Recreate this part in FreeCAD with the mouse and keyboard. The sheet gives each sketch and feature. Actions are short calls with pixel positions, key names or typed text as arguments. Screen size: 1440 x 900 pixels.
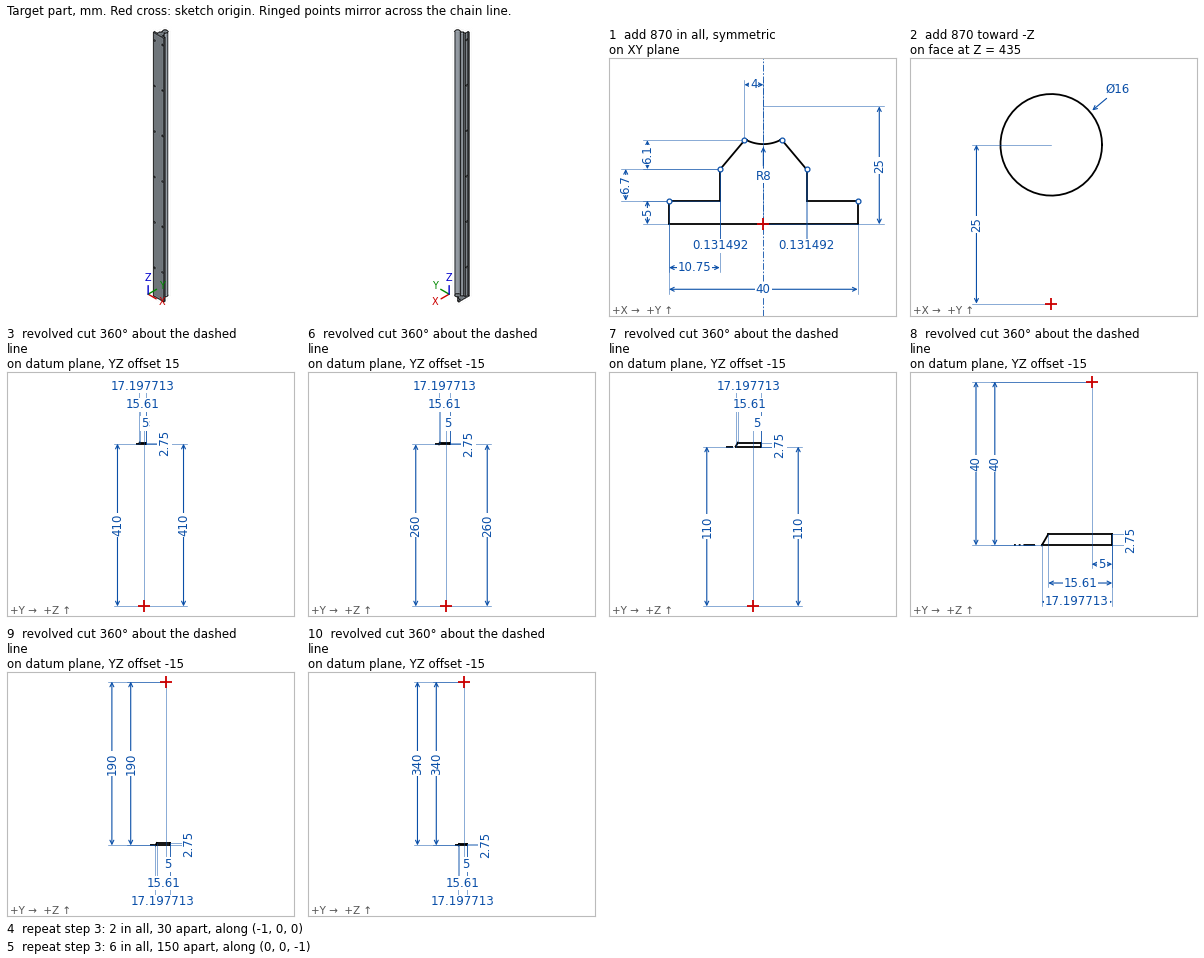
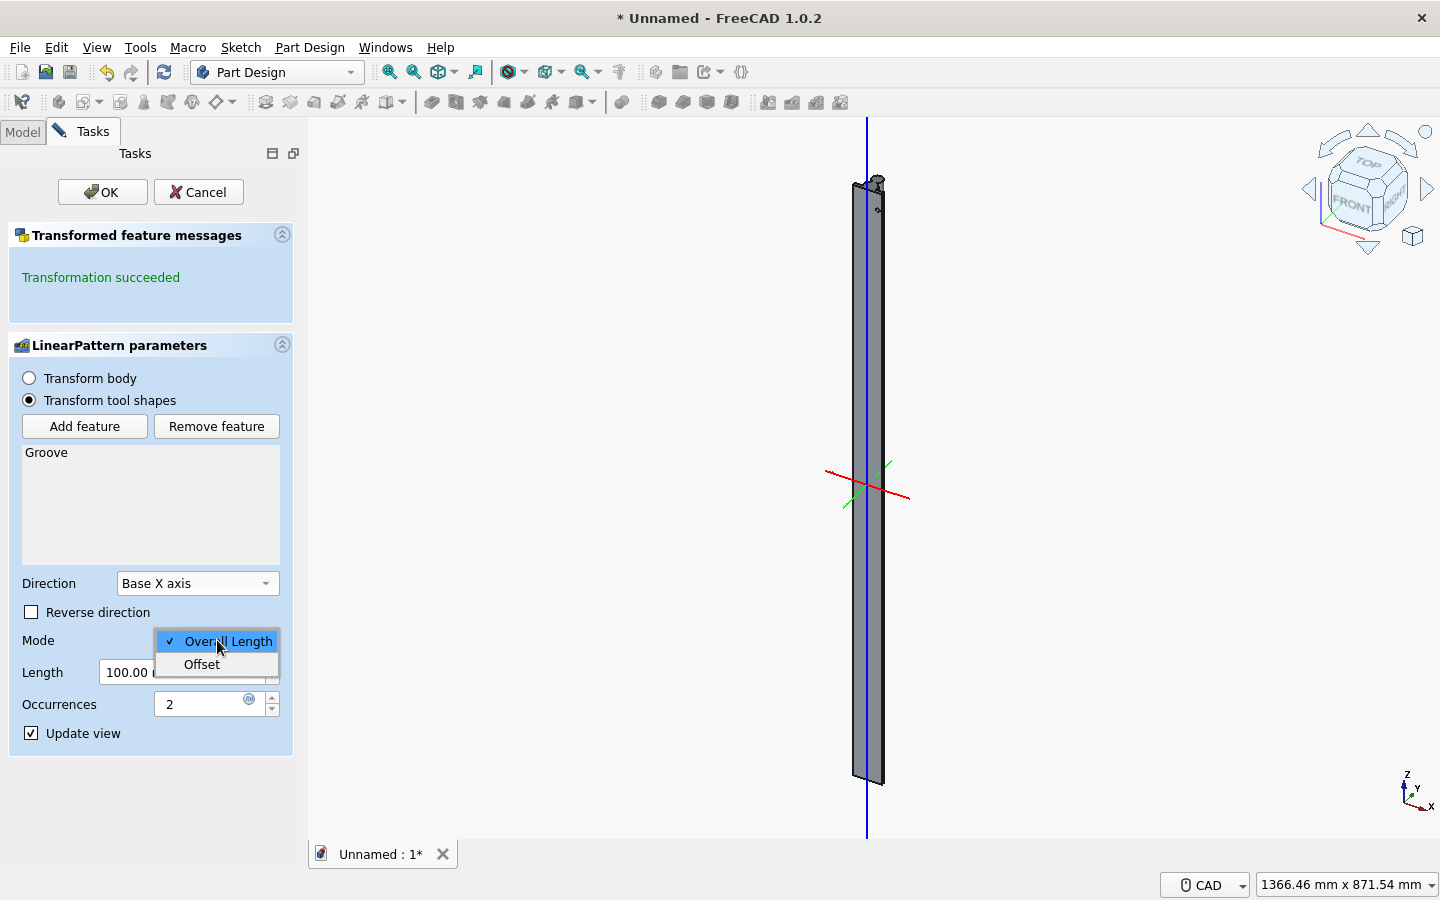
click(216, 664)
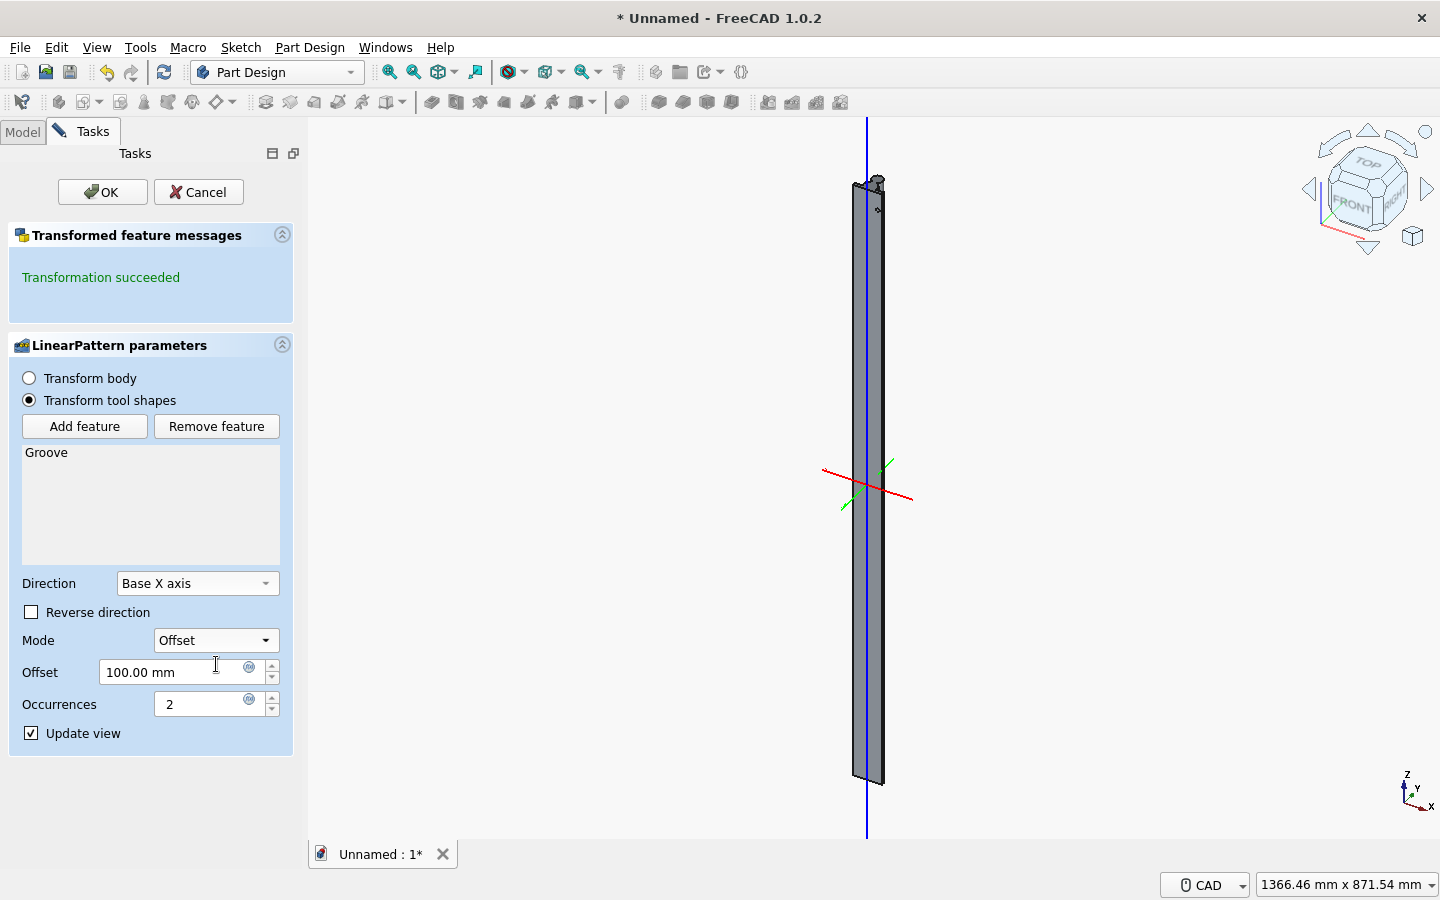
triple_click(182, 672)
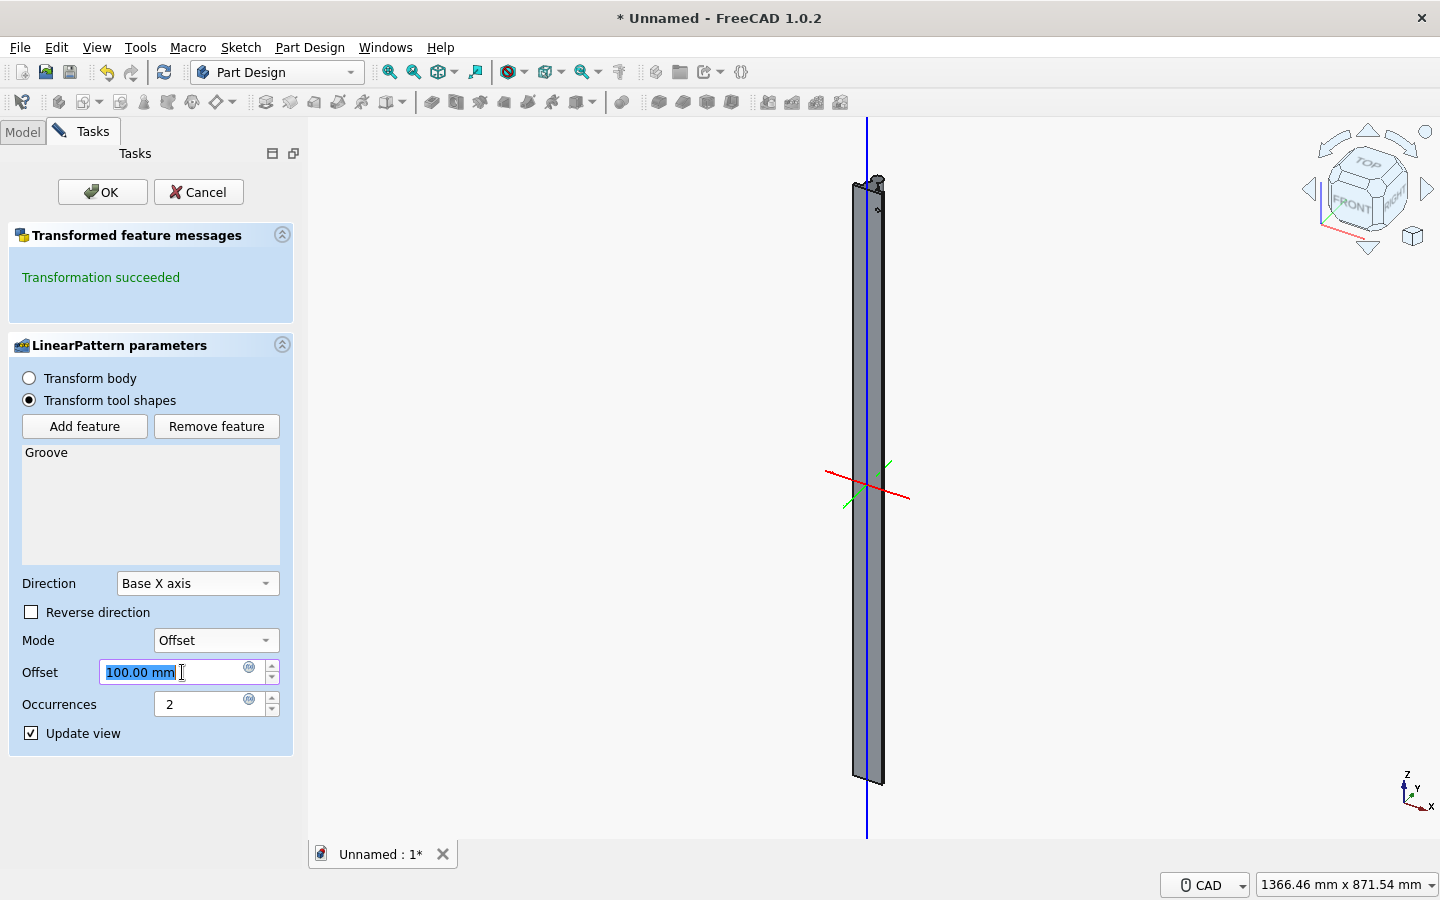
text(30)
key(Tab)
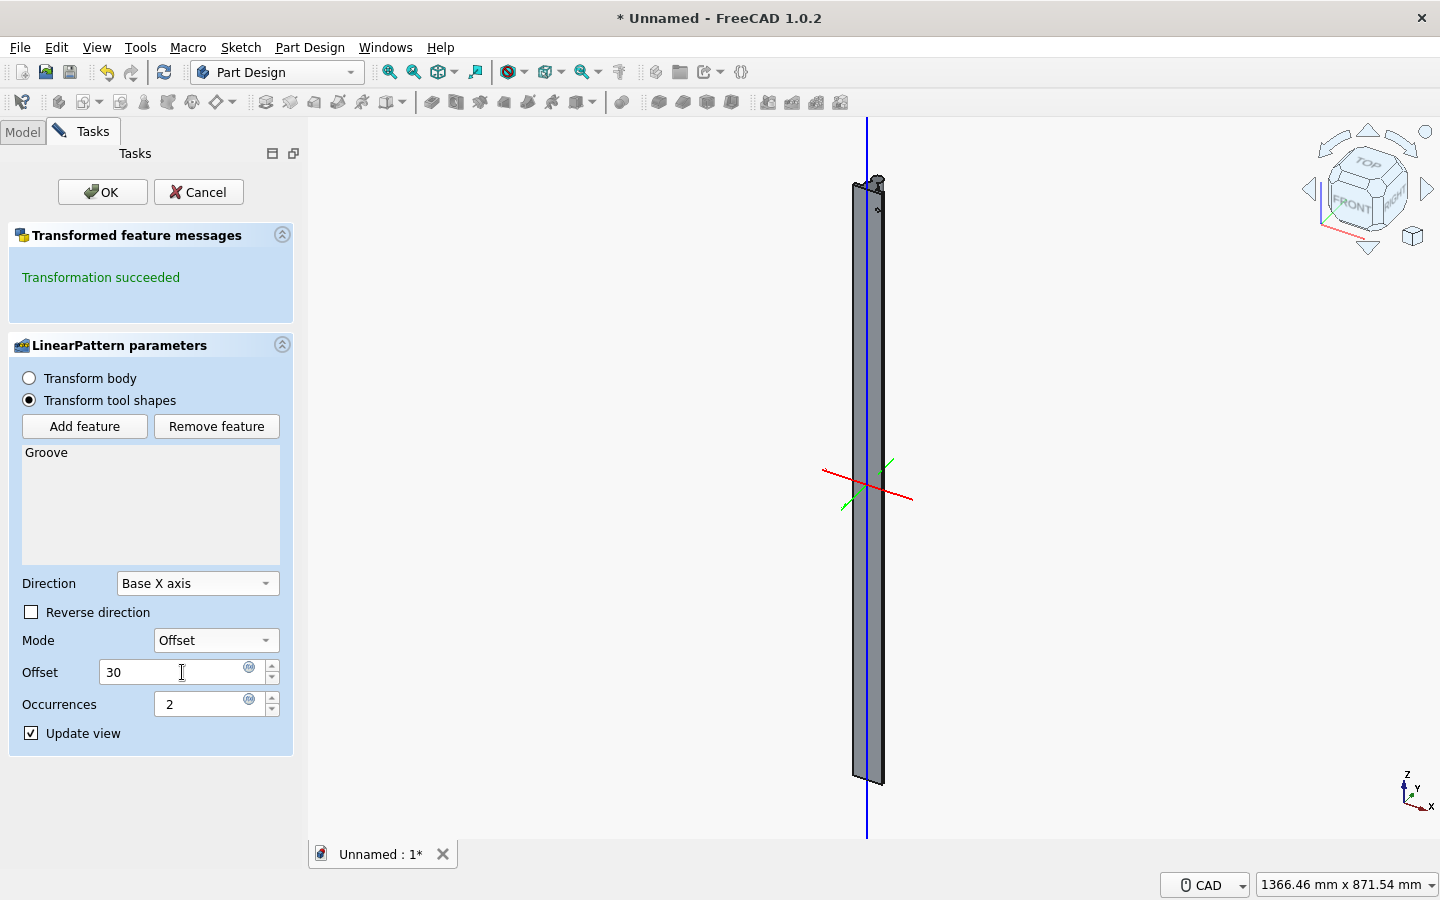
triple_click(209, 704)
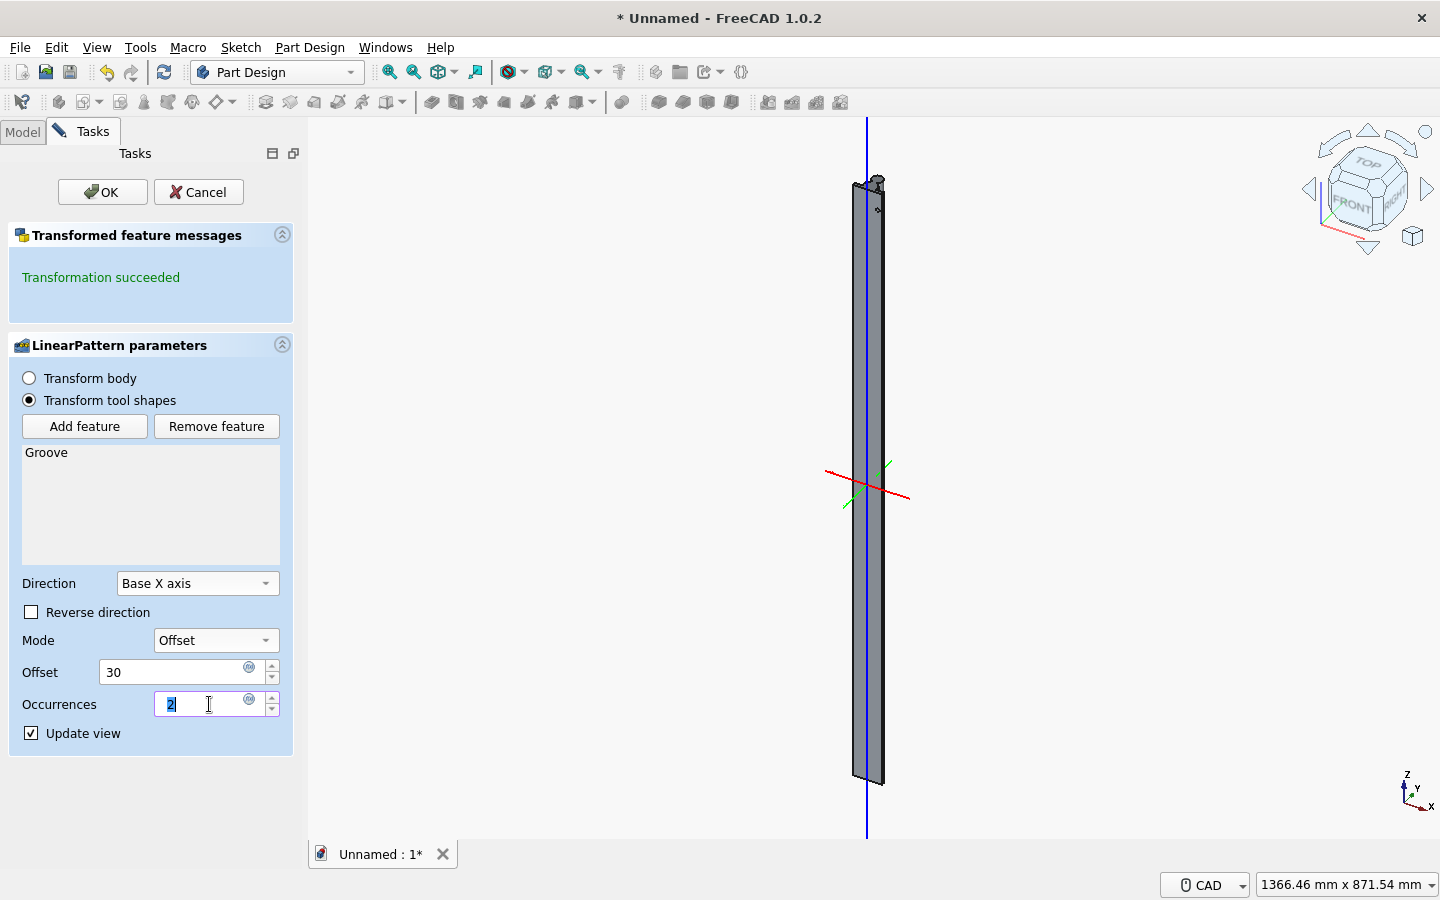
text(2)
key(Tab)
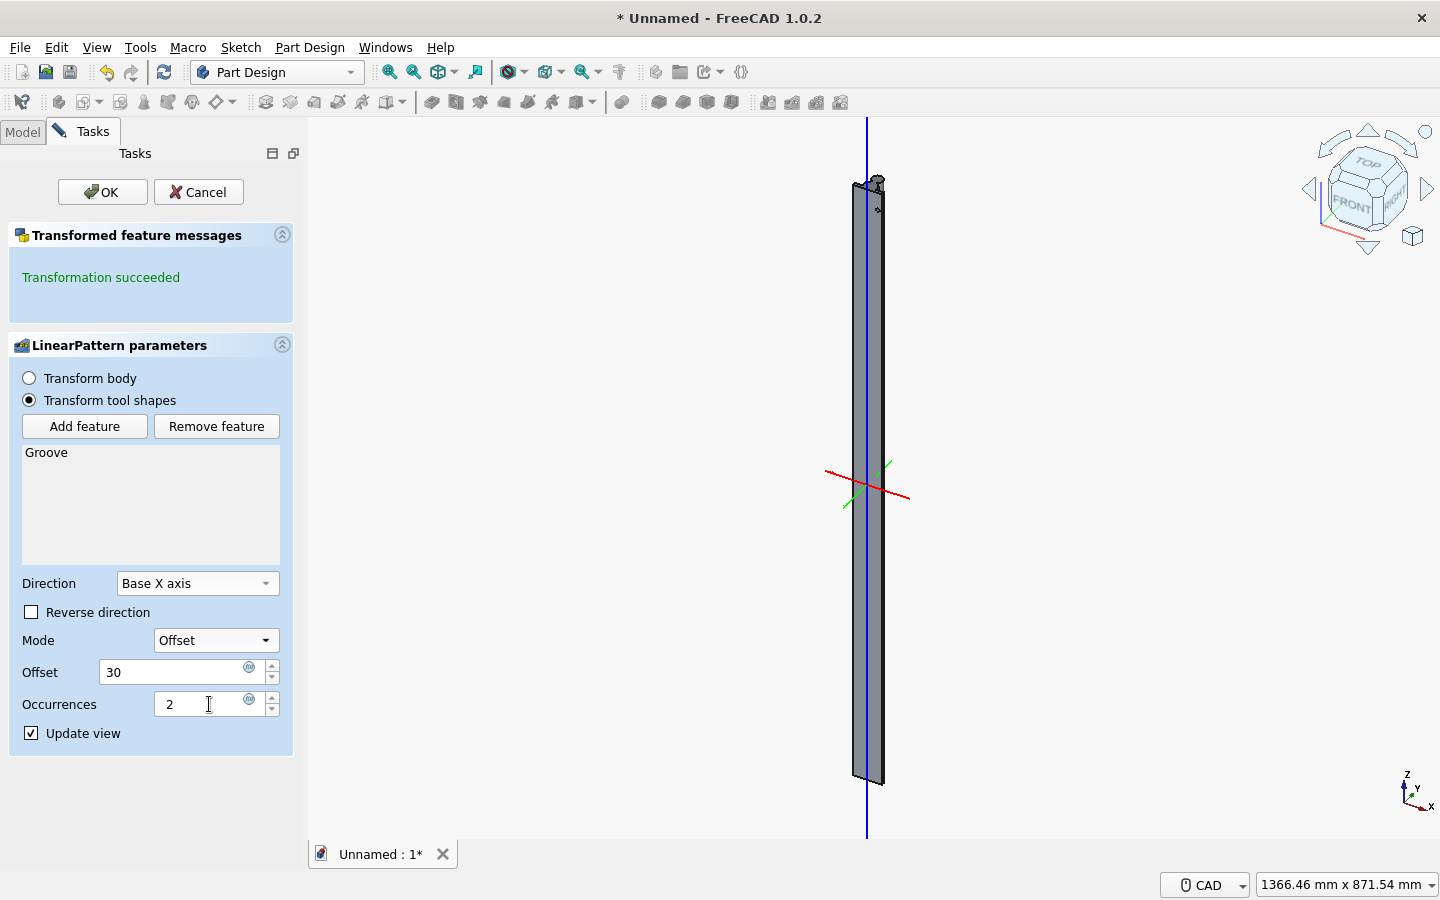
click(30, 612)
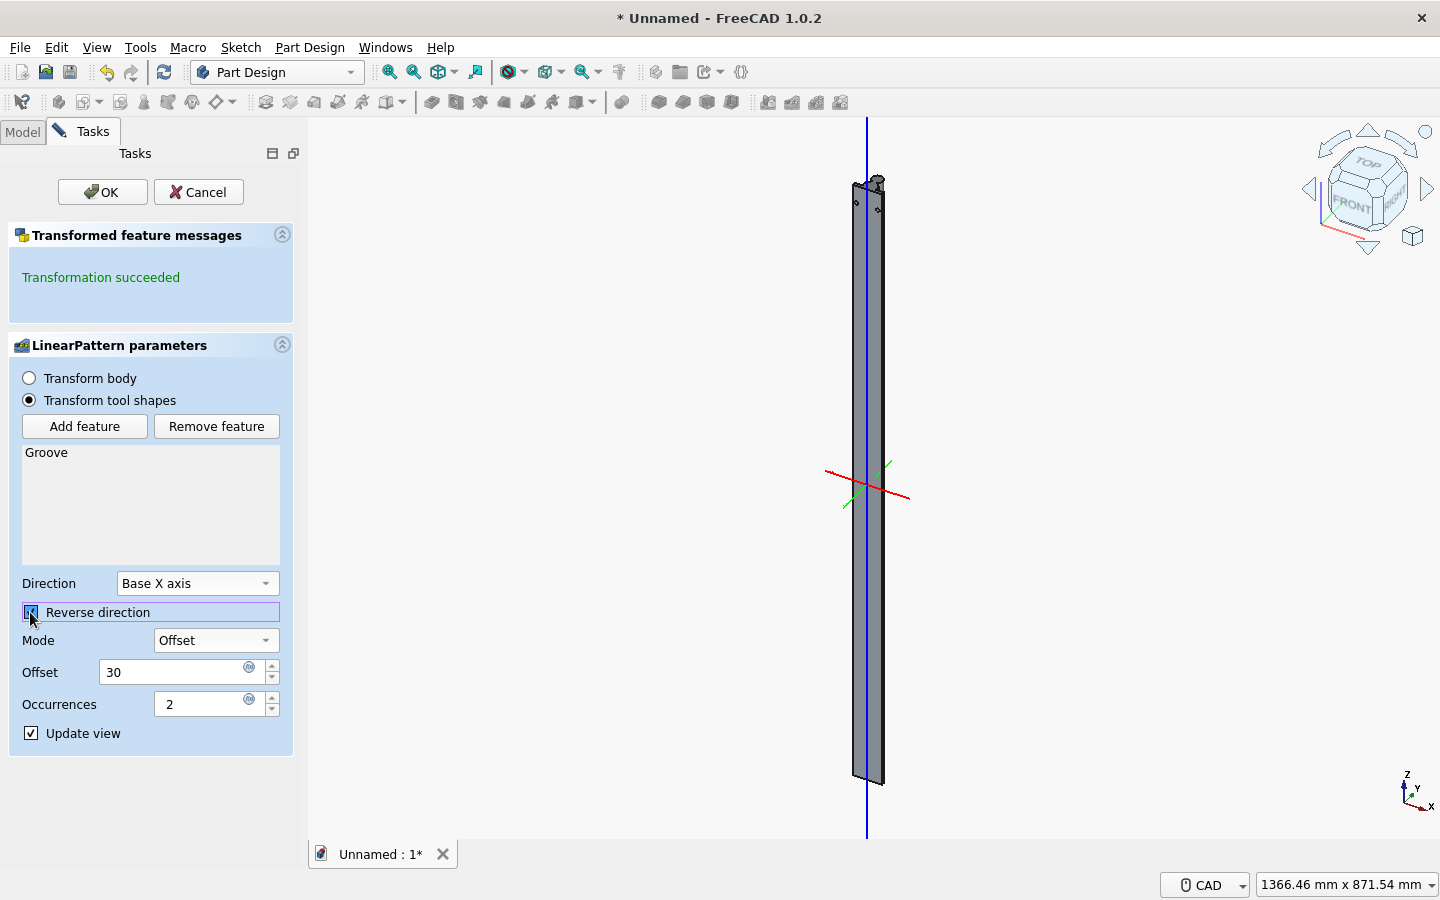
click(103, 192)